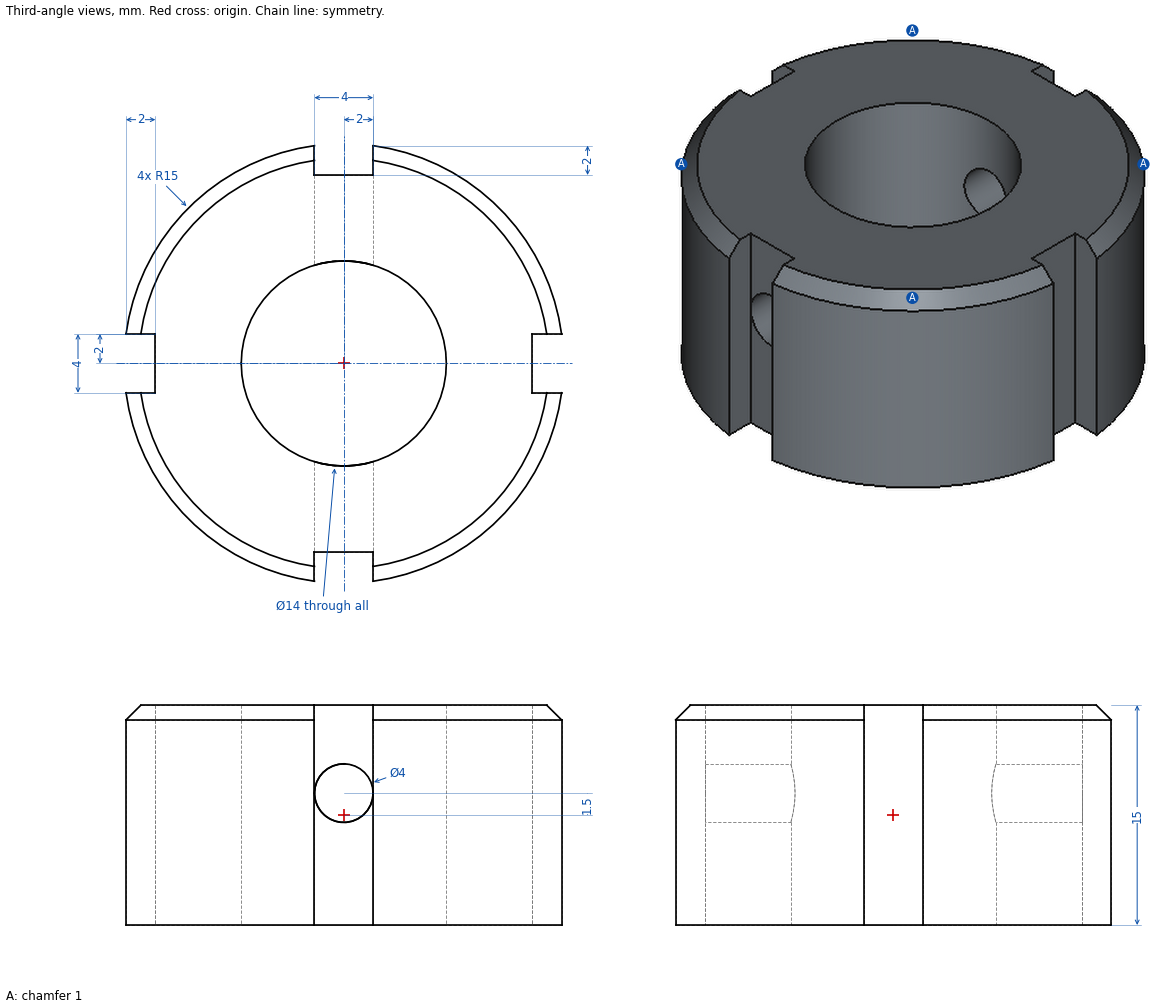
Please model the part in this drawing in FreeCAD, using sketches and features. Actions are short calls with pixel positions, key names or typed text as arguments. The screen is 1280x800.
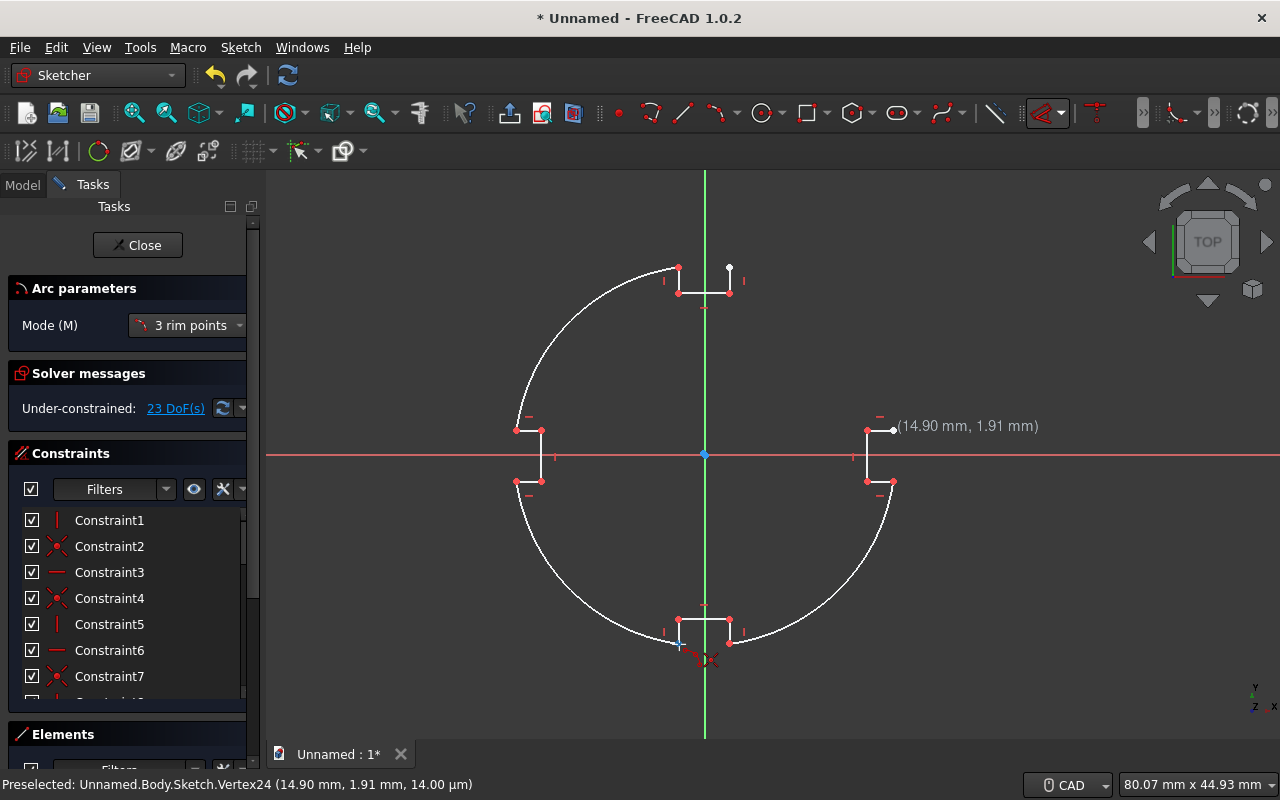
scroll(730, 267, up, 2)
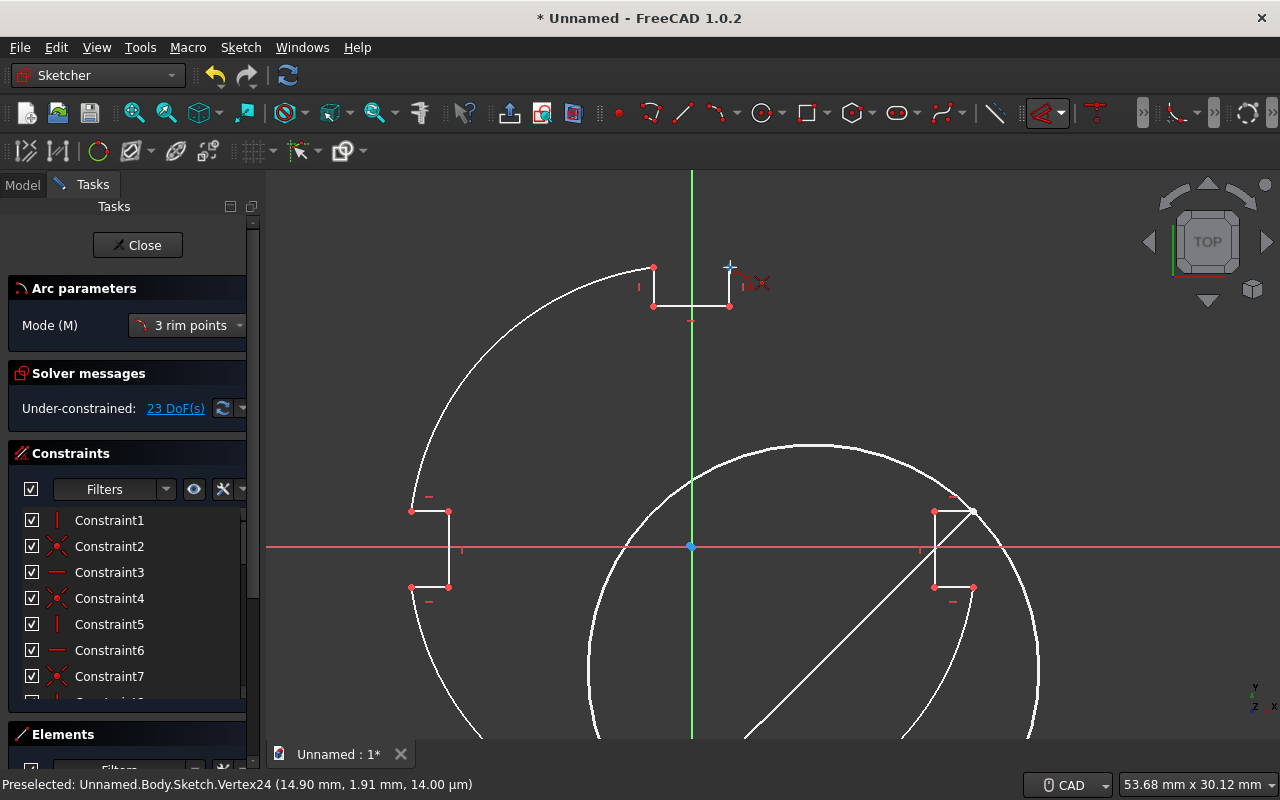
click(729, 267)
click(892, 347)
key(Escape)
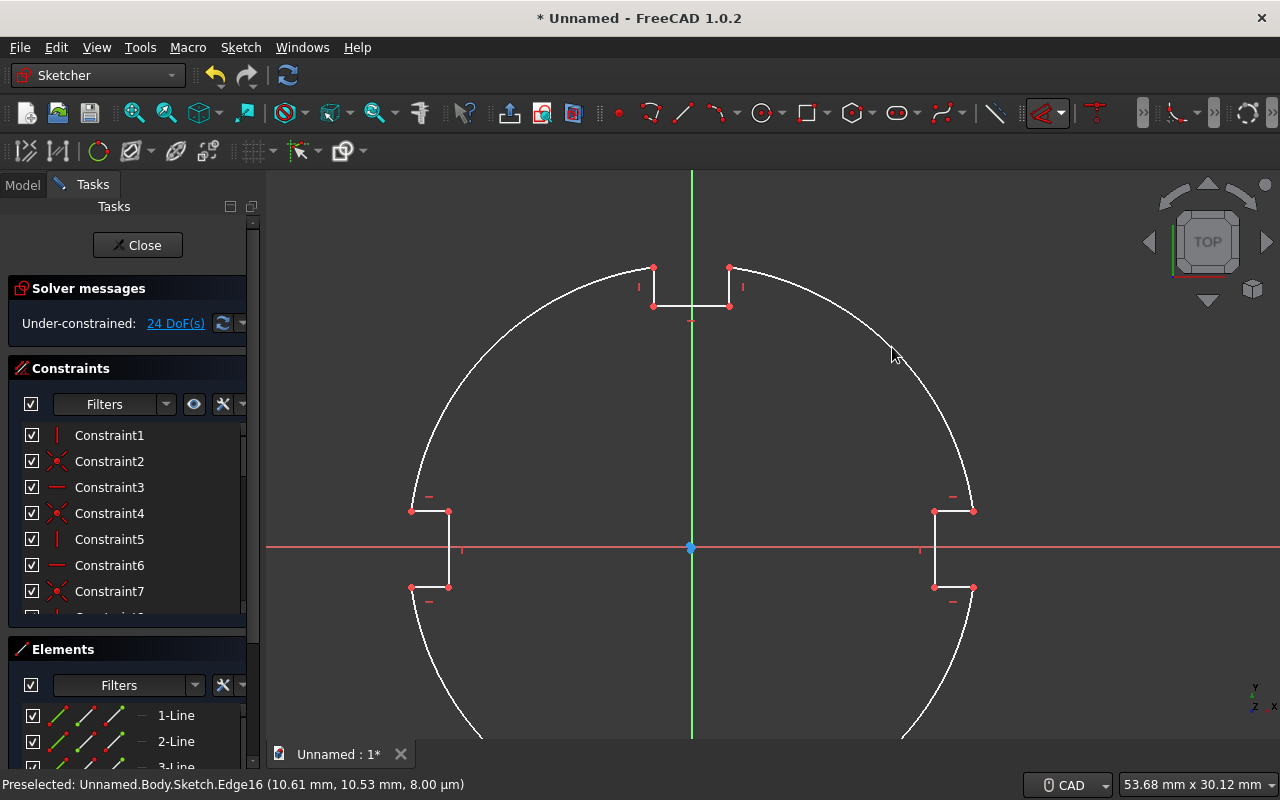
click(549, 303)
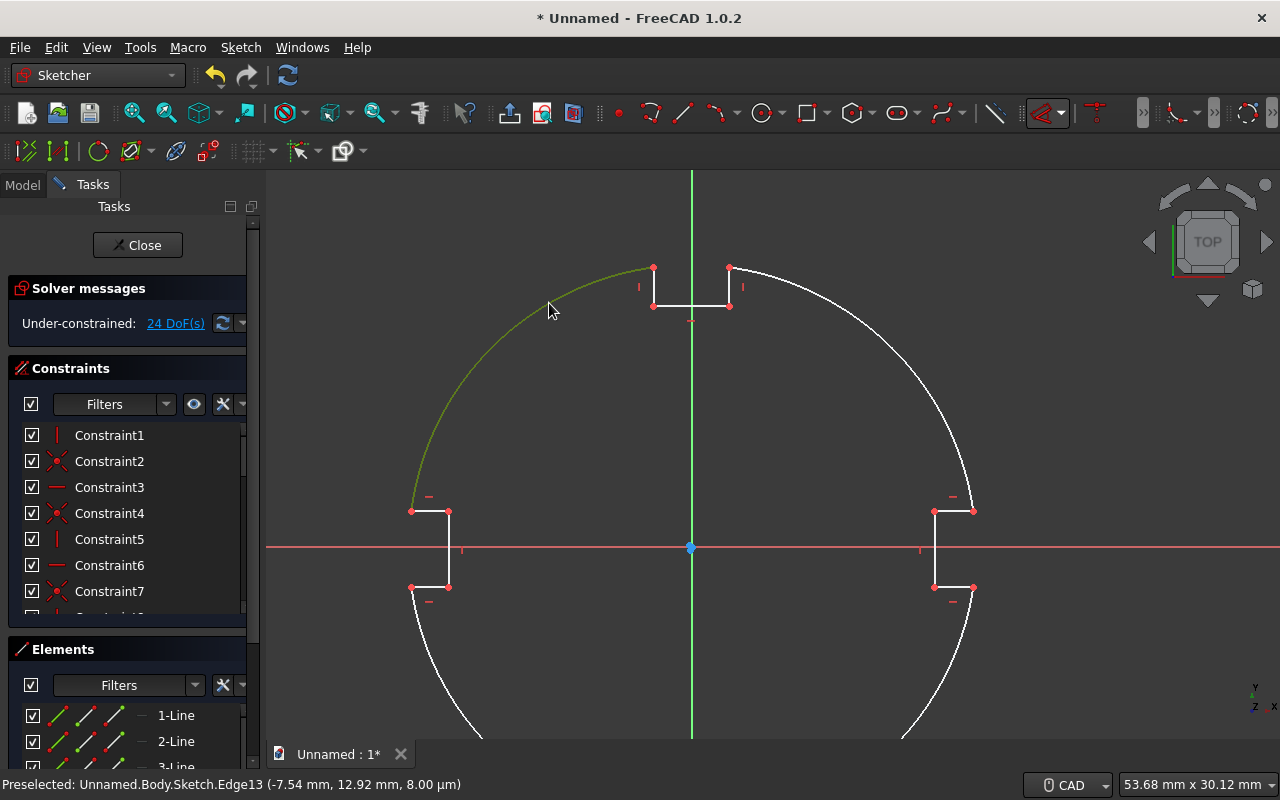
click(447, 691)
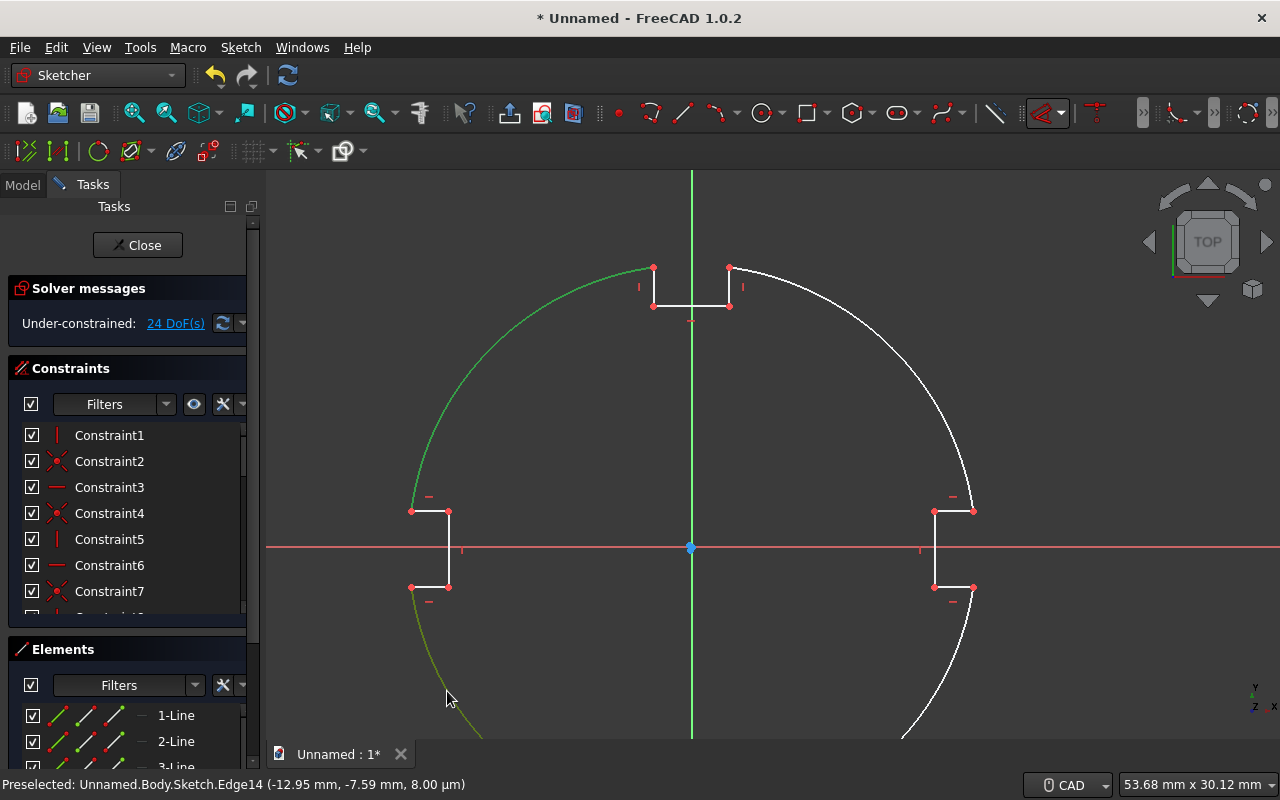
key(c)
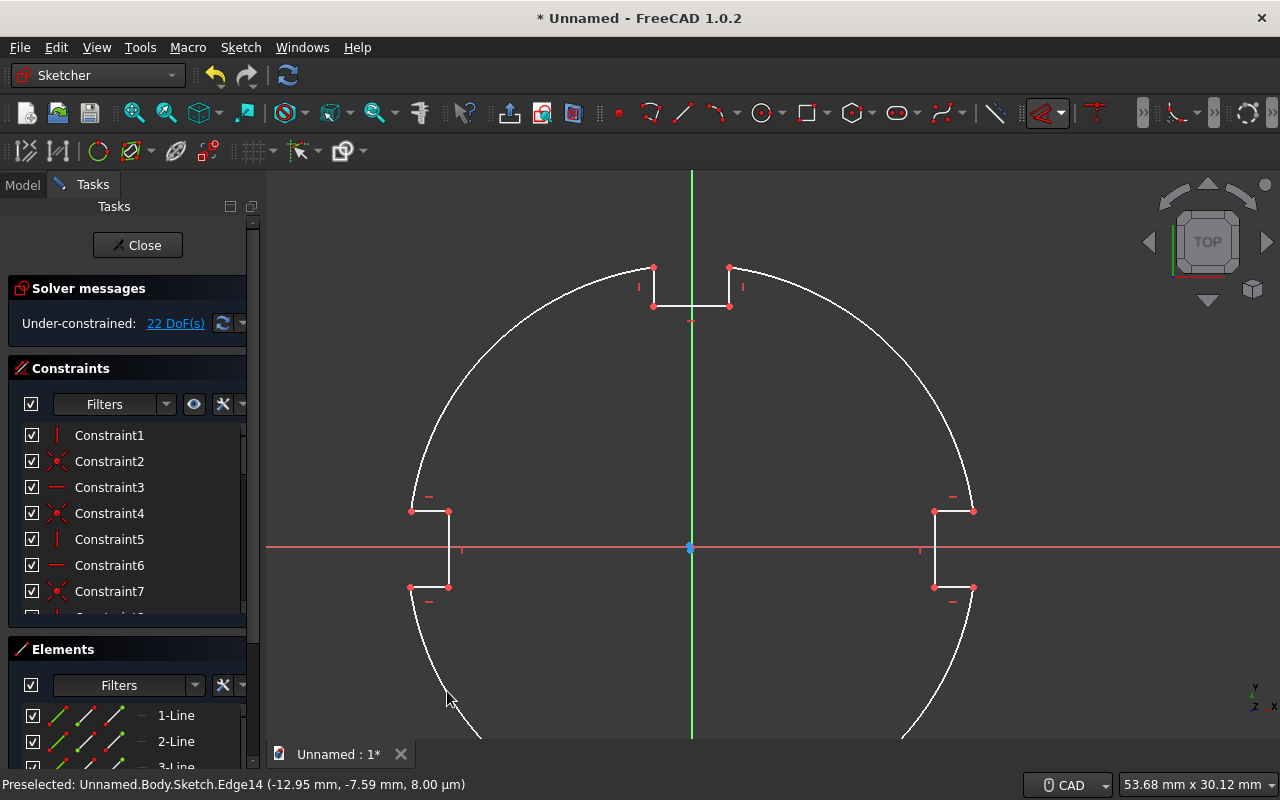
click(549, 303)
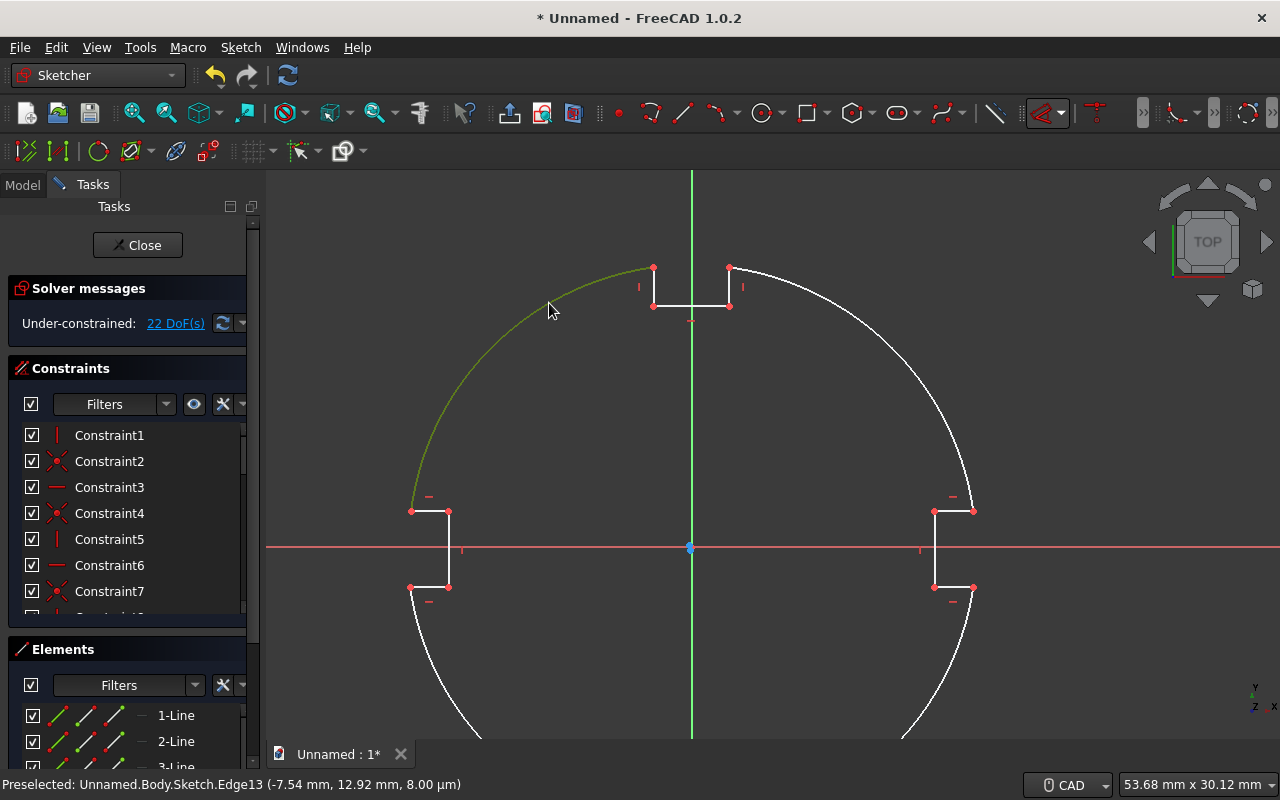
click(937, 691)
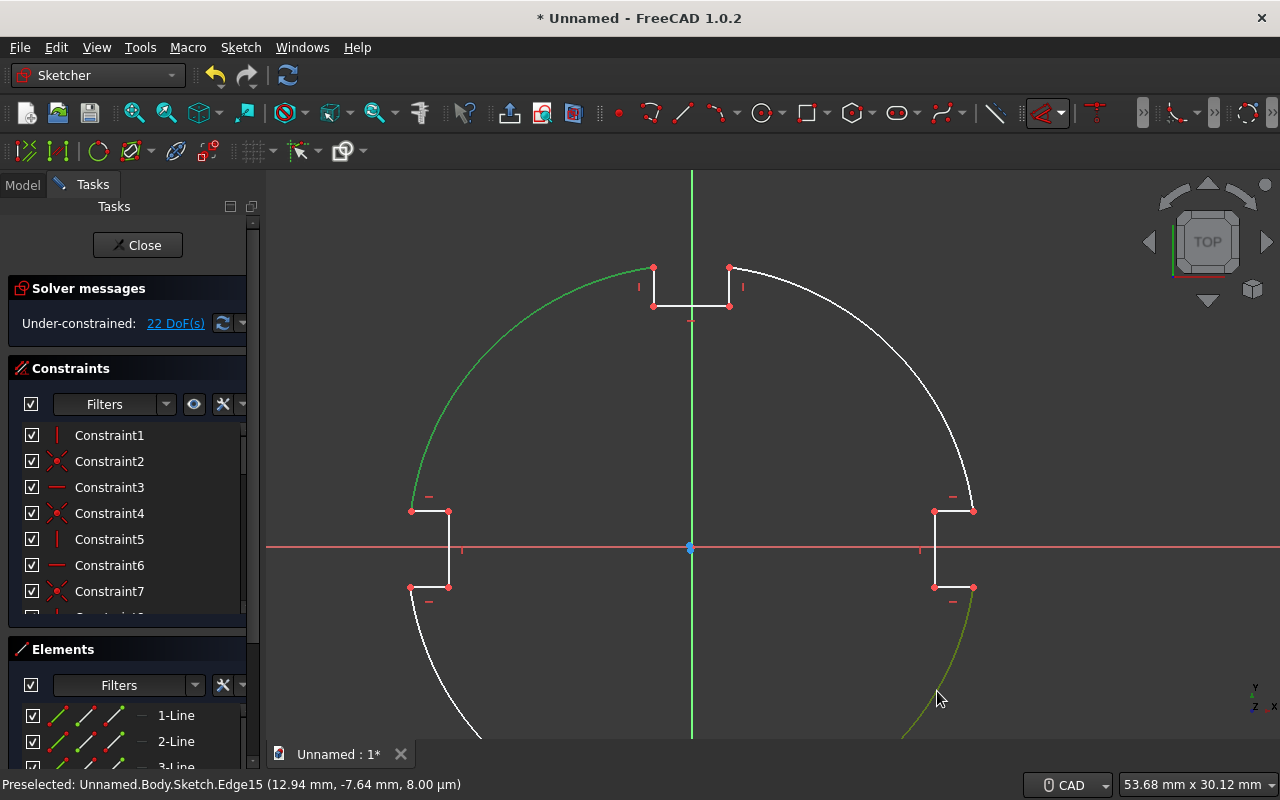
key(c)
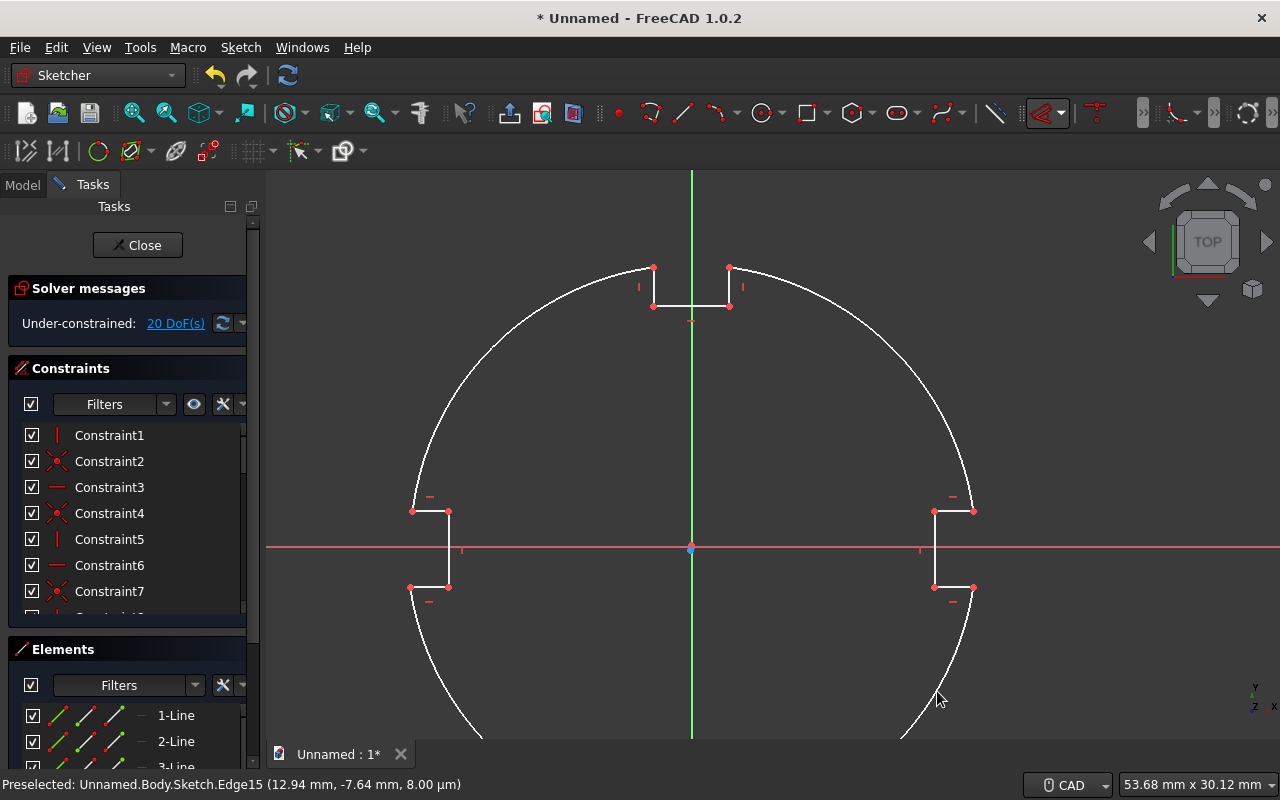
click(550, 303)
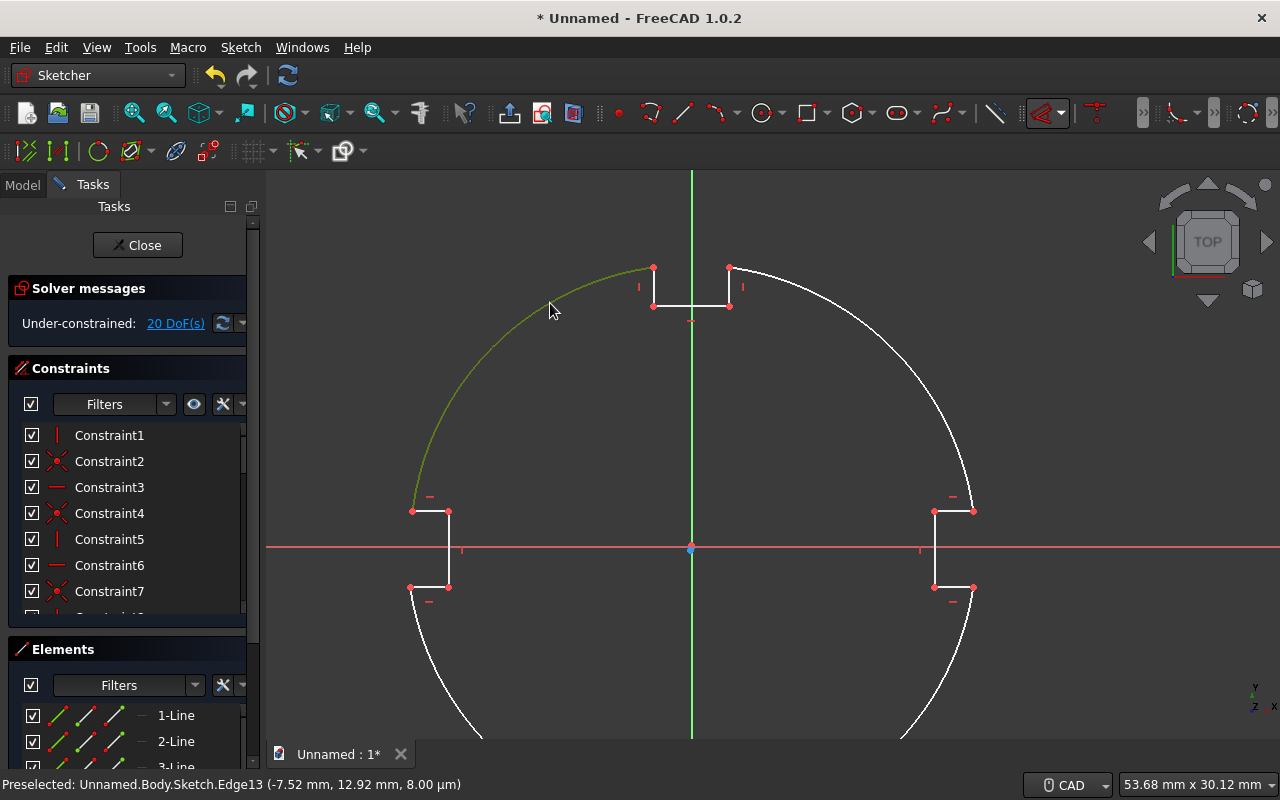
click(937, 407)